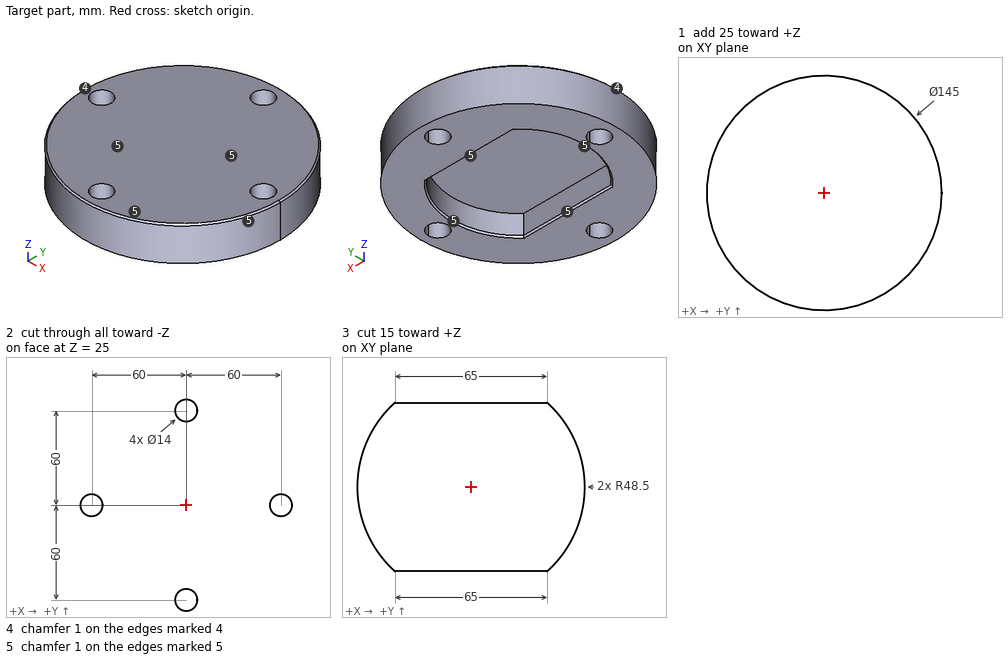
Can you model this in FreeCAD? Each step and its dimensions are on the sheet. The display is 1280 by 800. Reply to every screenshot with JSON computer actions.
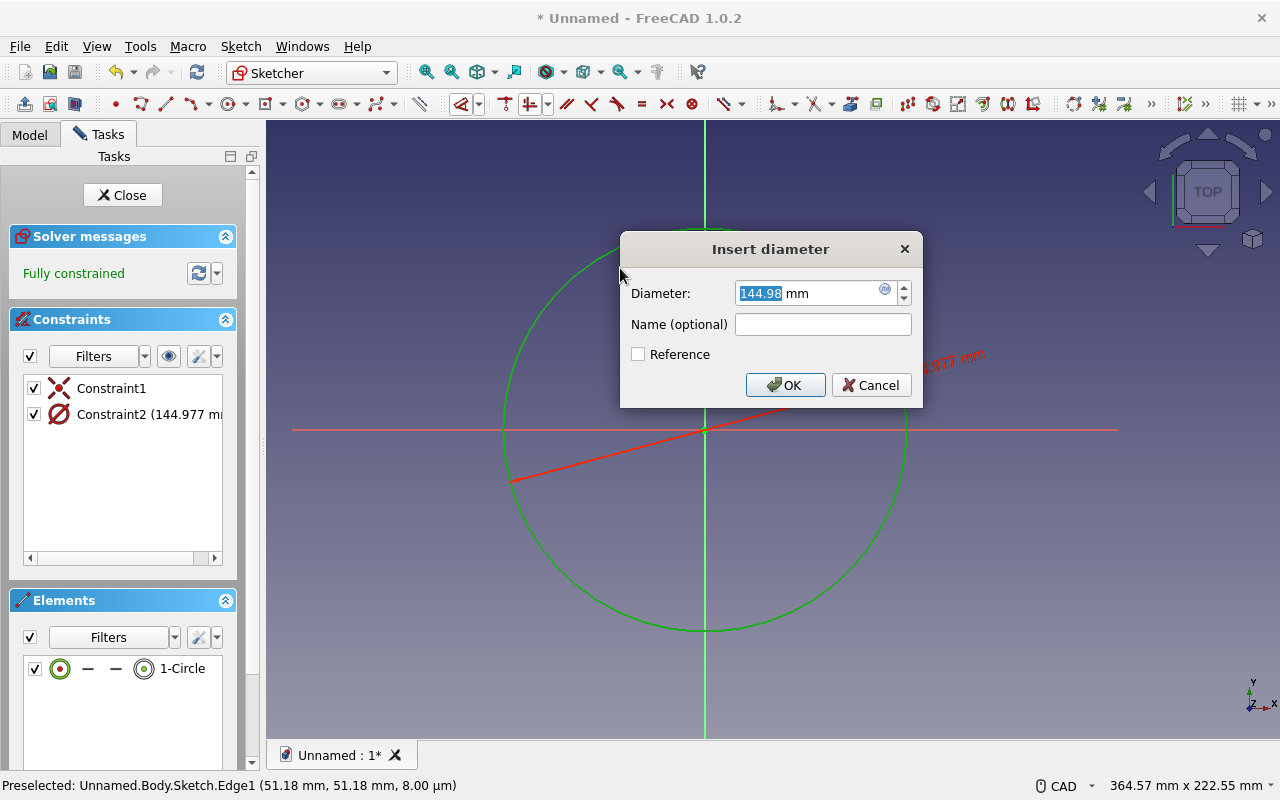
{"action": "type", "text": "145"}
{"action": "key", "text": "Return"}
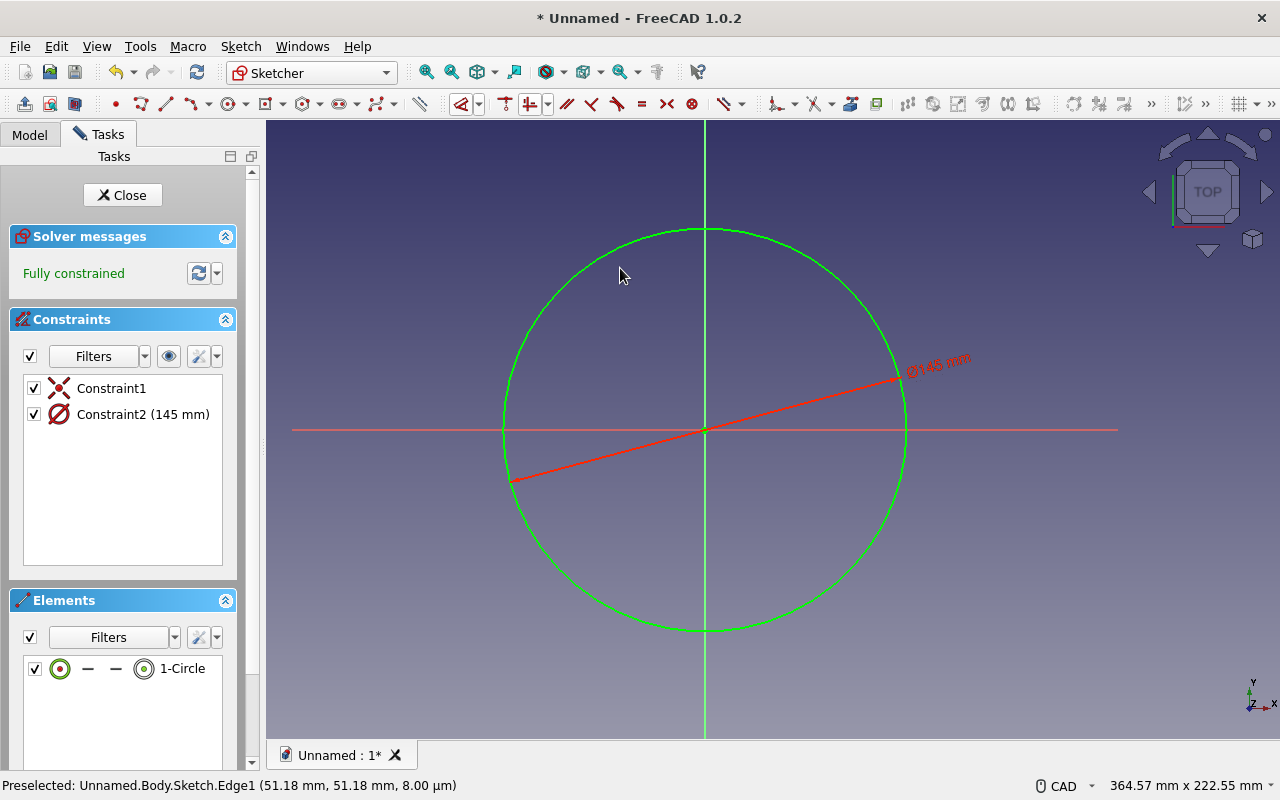
{"action": "left_click", "coordinate": [123, 195]}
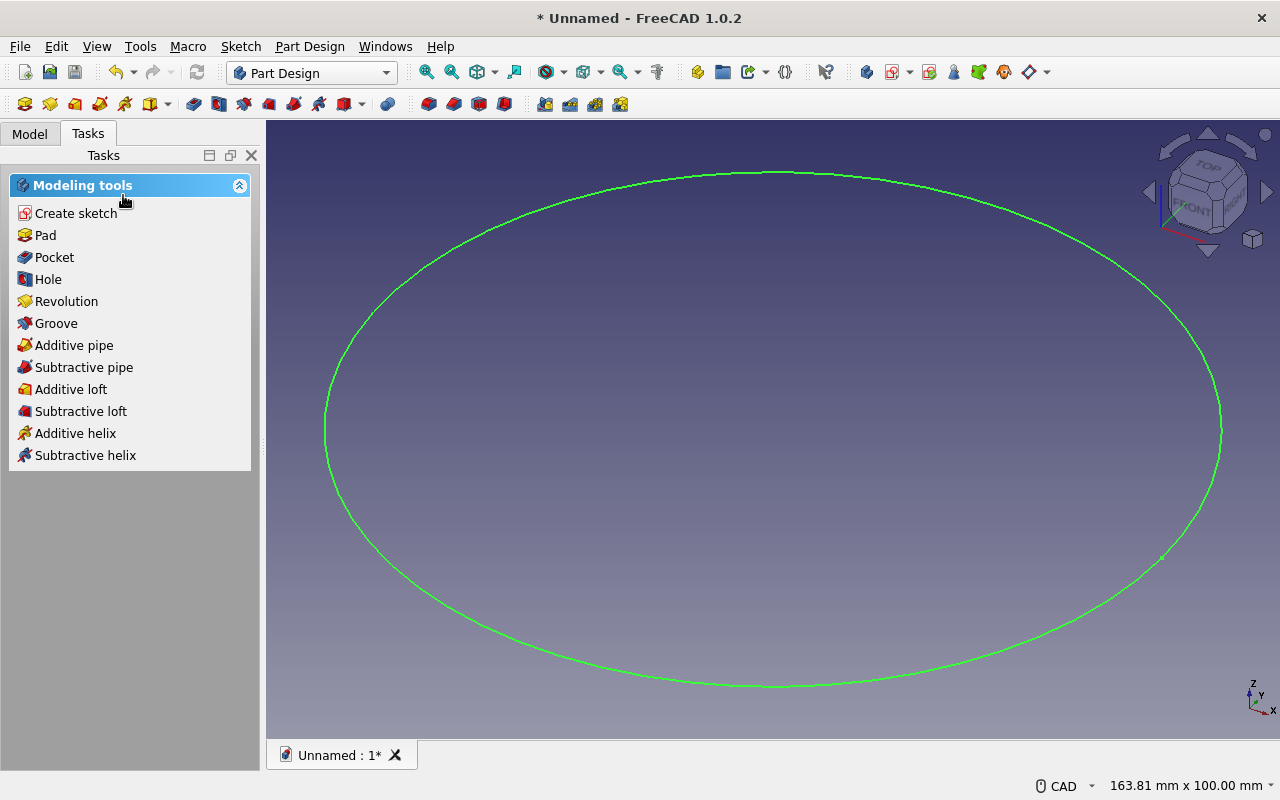
{"action": "left_click", "coordinate": [25, 104]}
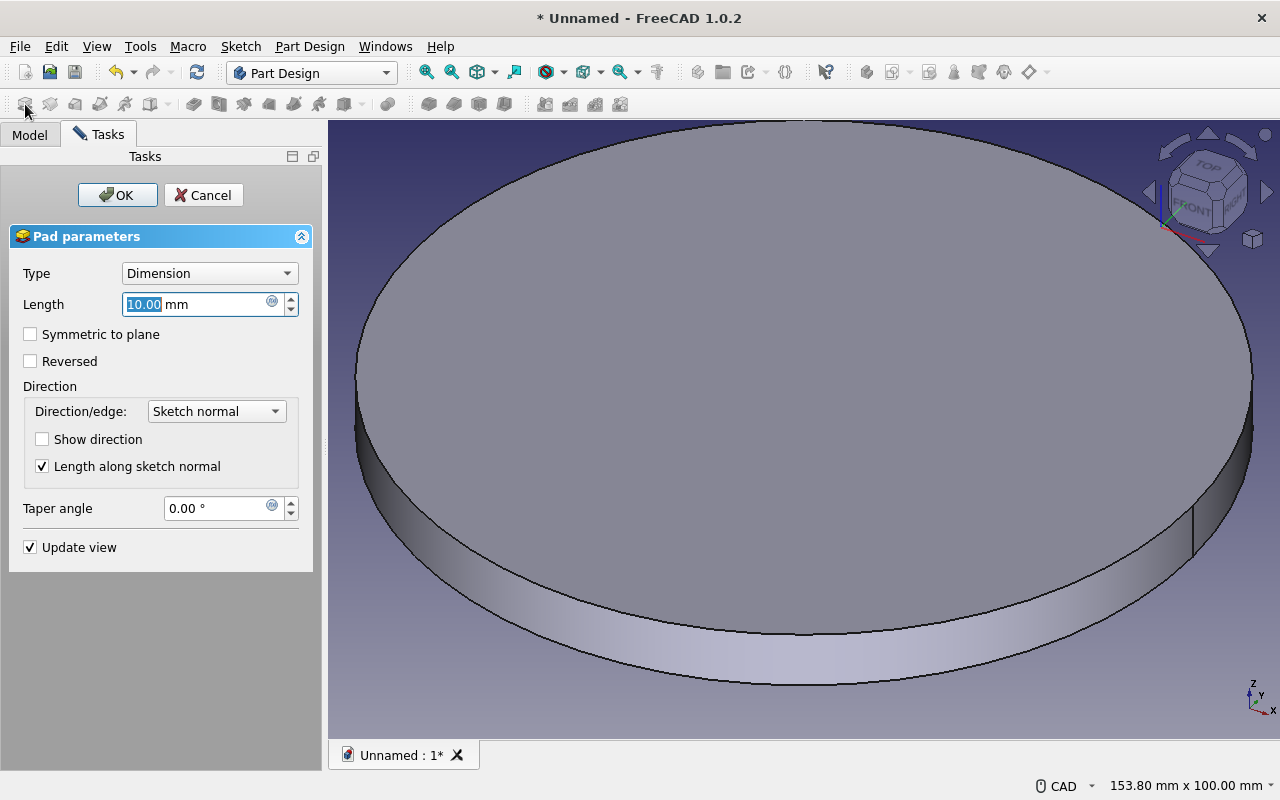
{"action": "type", "text": "25"}
{"action": "key", "text": "Tab"}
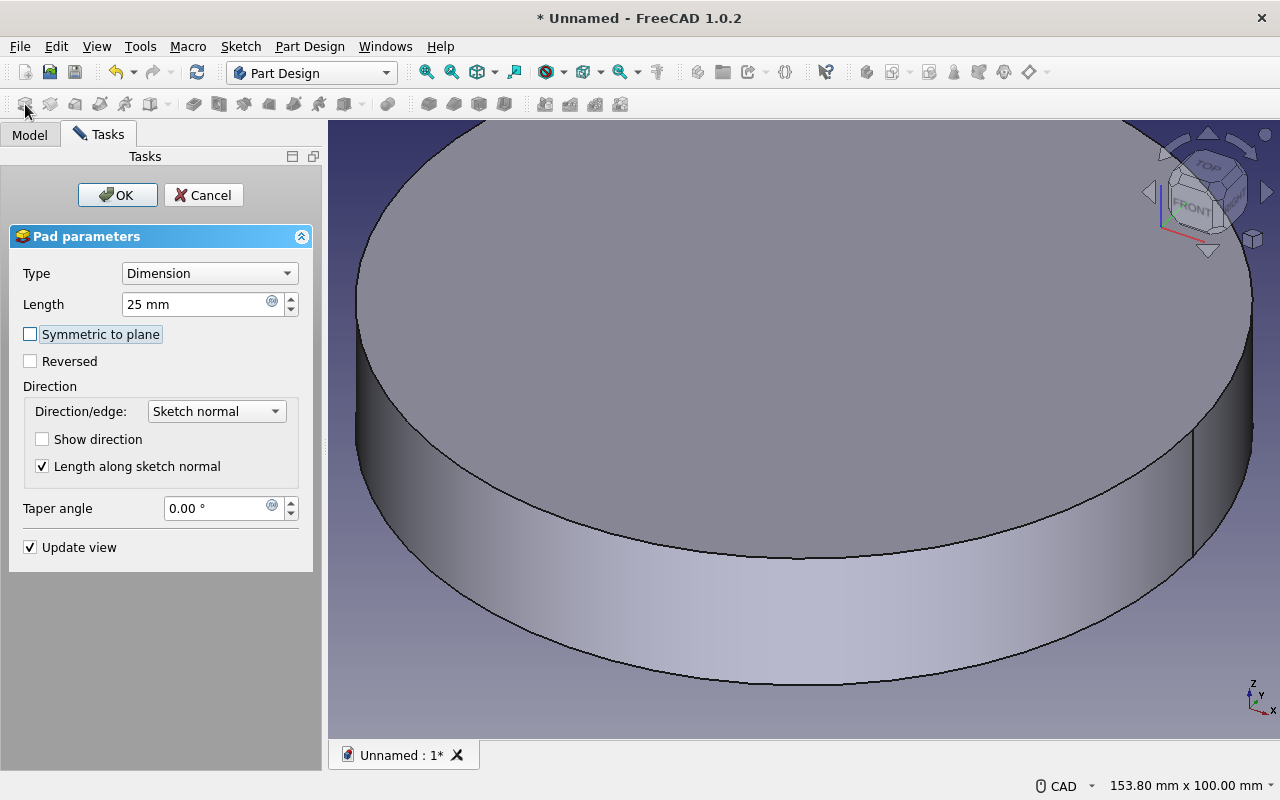
{"action": "left_click", "coordinate": [118, 195]}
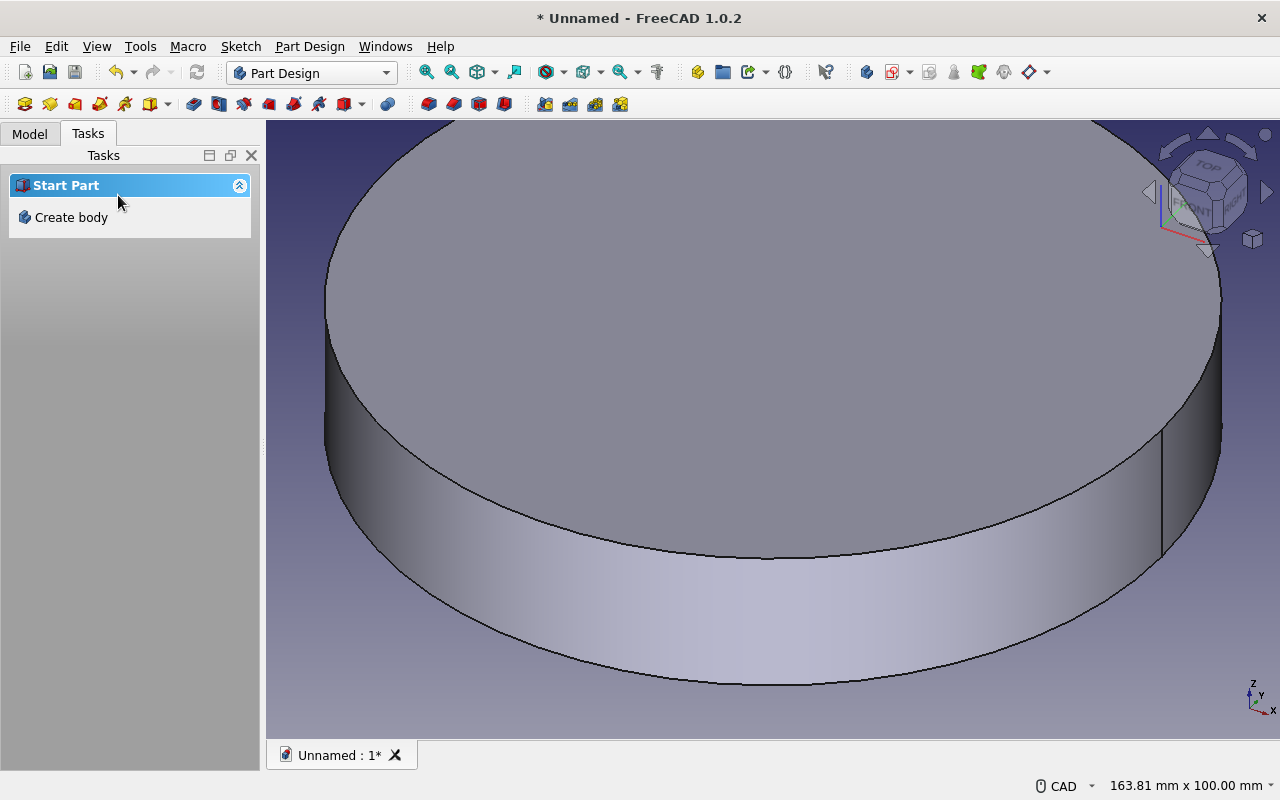
{"action": "left_click", "coordinate": [427, 72]}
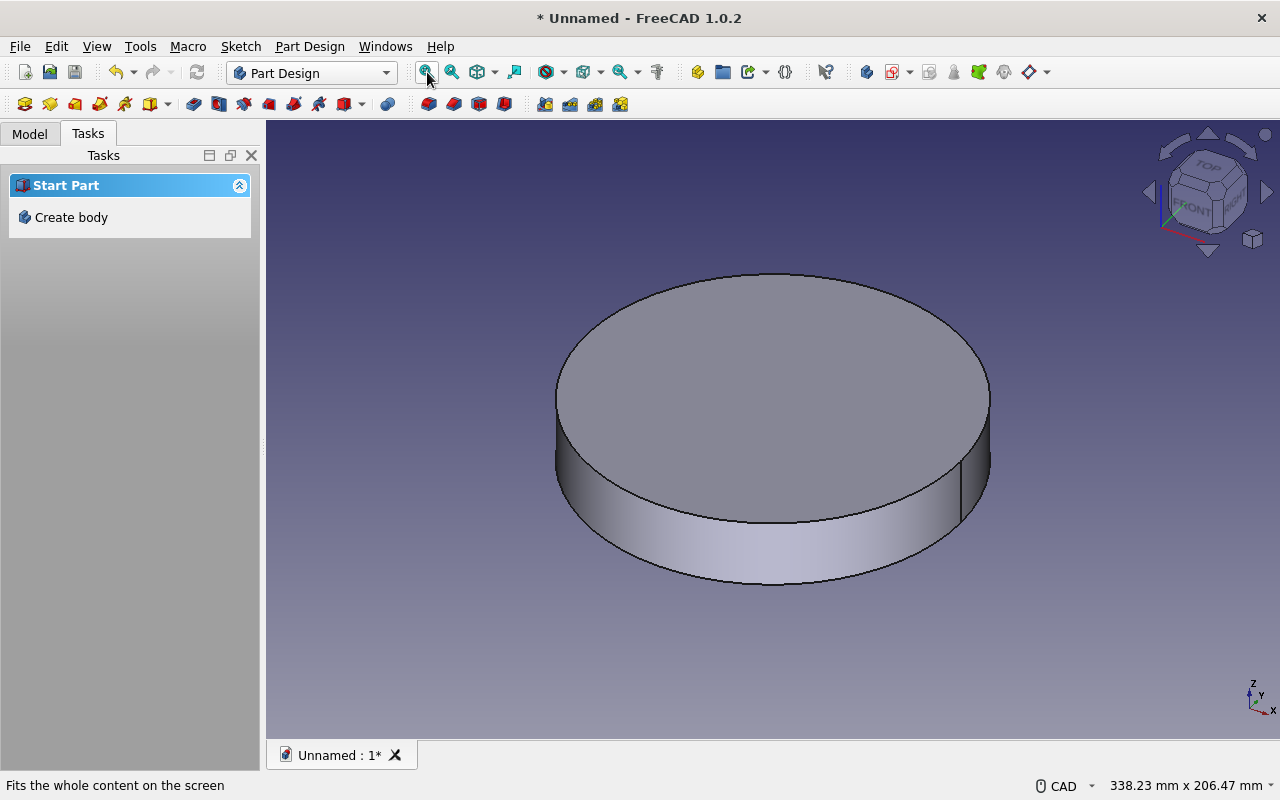
{"action": "left_click", "coordinate": [773, 398]}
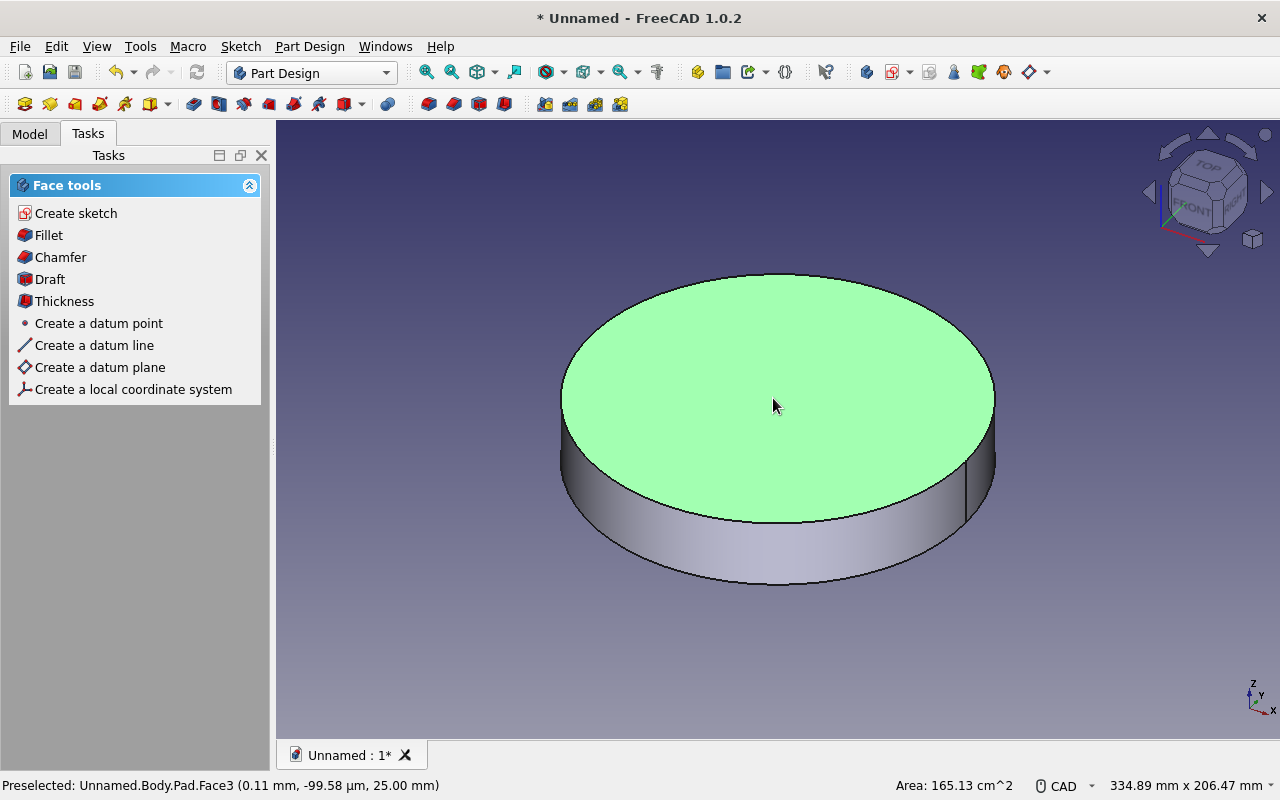
{"action": "left_click", "coordinate": [892, 72]}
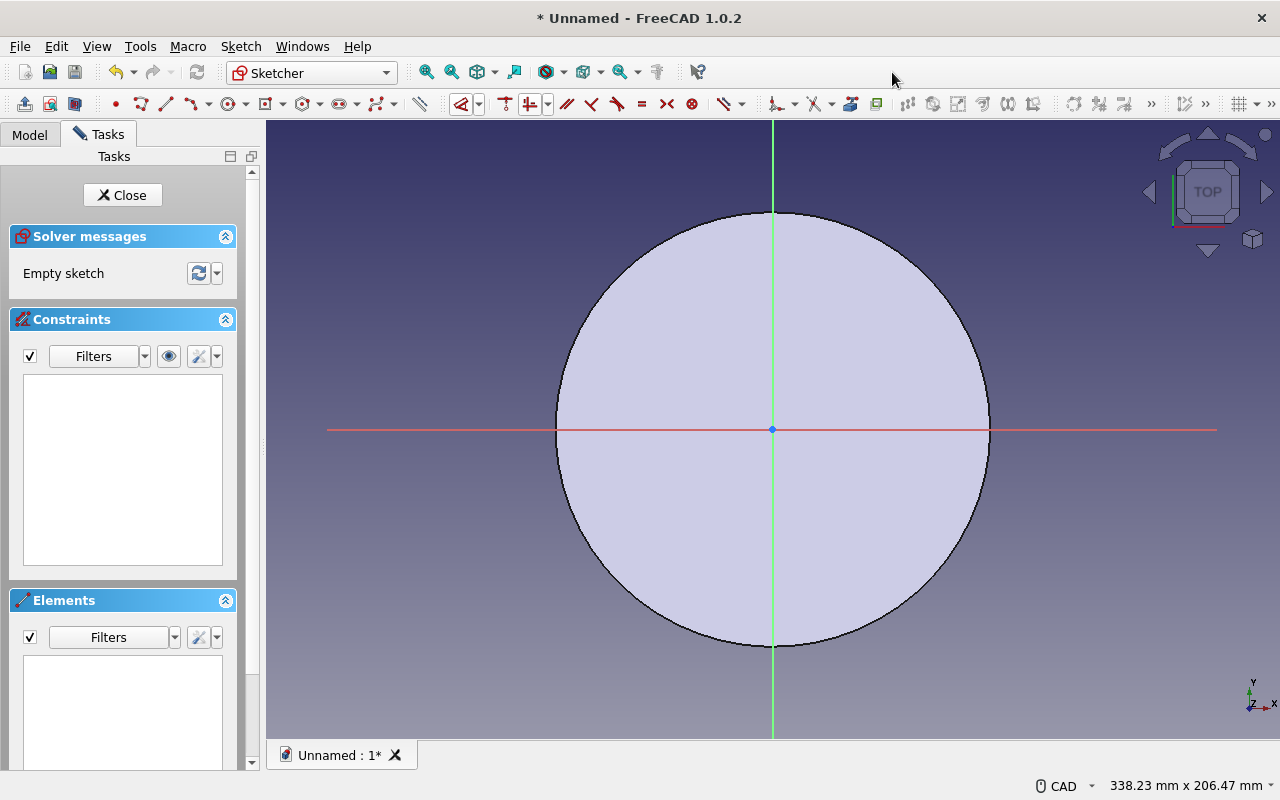
{"action": "left_click", "coordinate": [228, 104]}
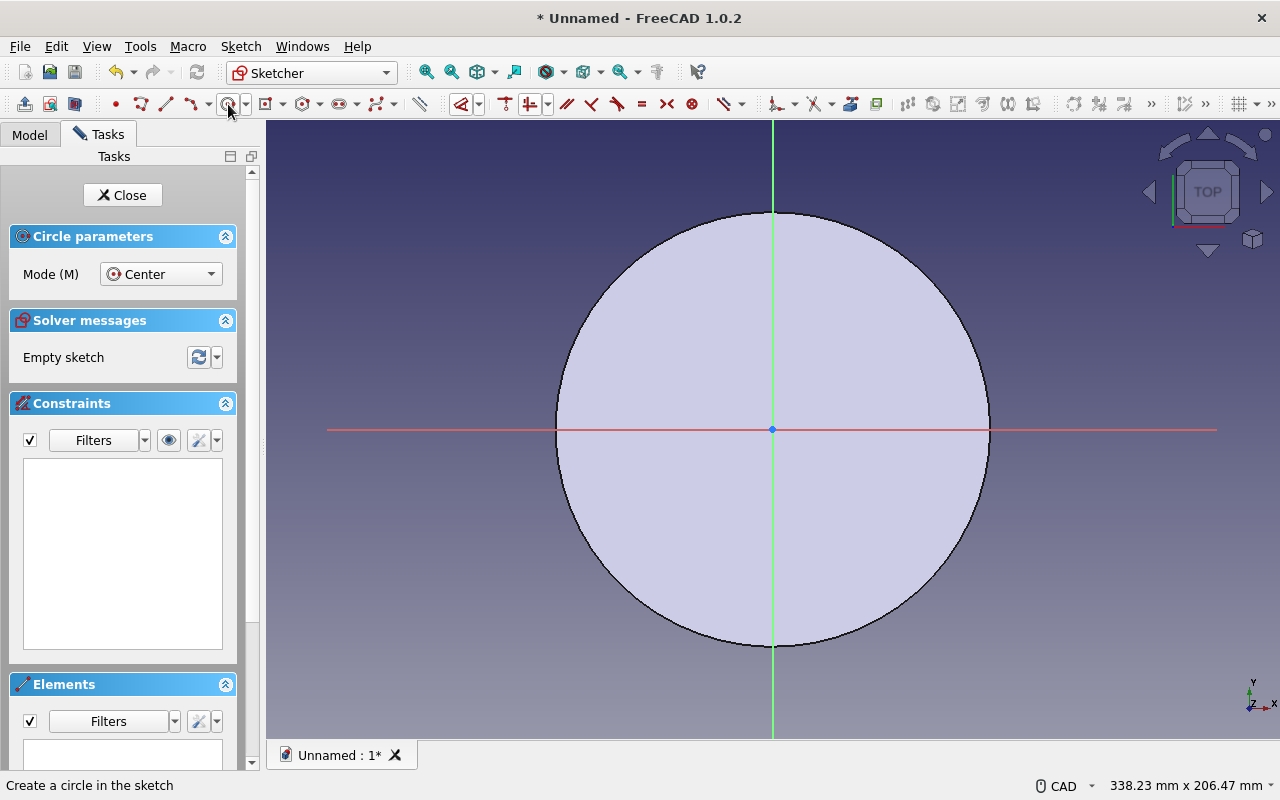
{"action": "left_click", "coordinate": [773, 250]}
{"action": "left_click", "coordinate": [788, 235]}